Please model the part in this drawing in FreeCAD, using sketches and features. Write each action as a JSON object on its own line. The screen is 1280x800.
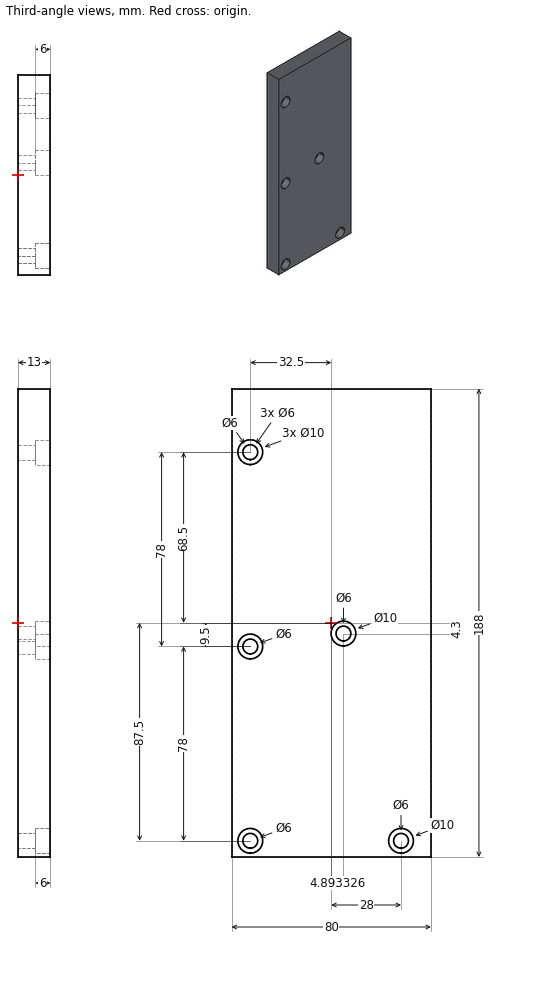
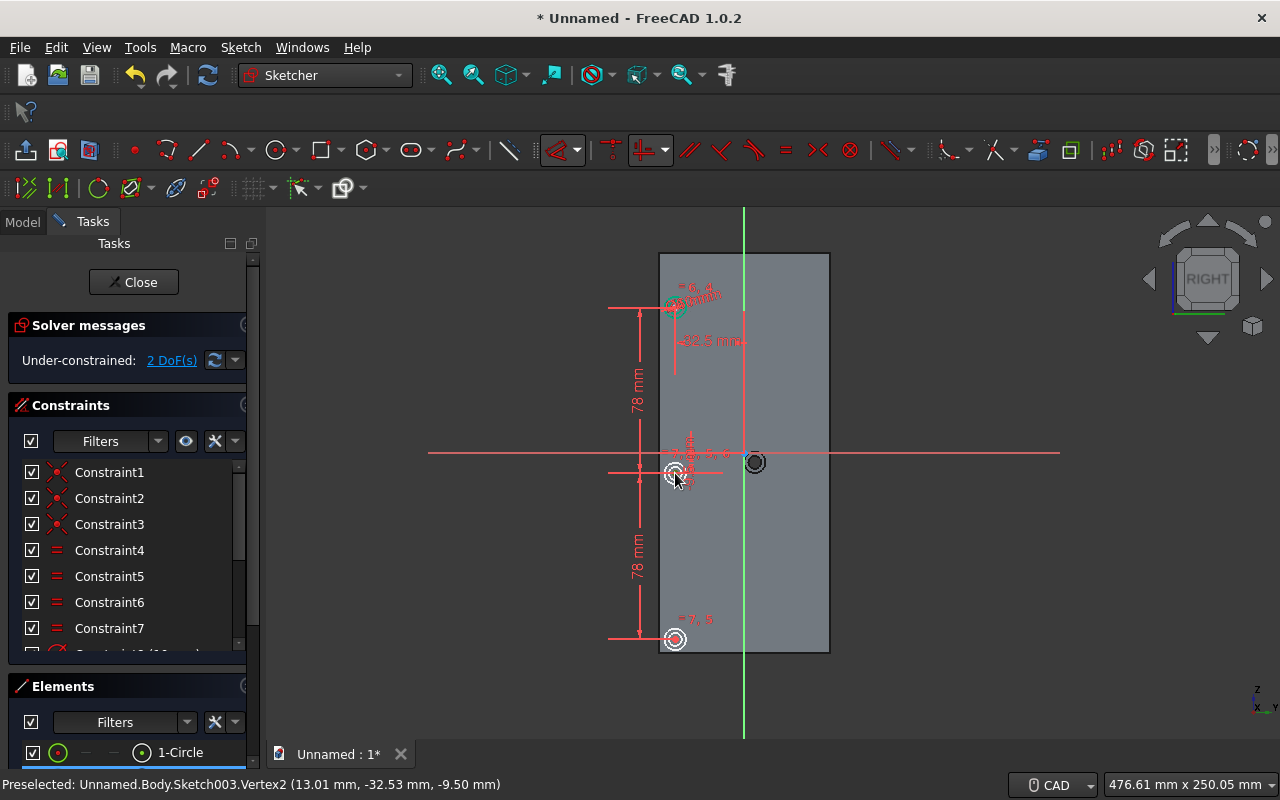
{"action": "left_click", "coordinate": [580, 150]}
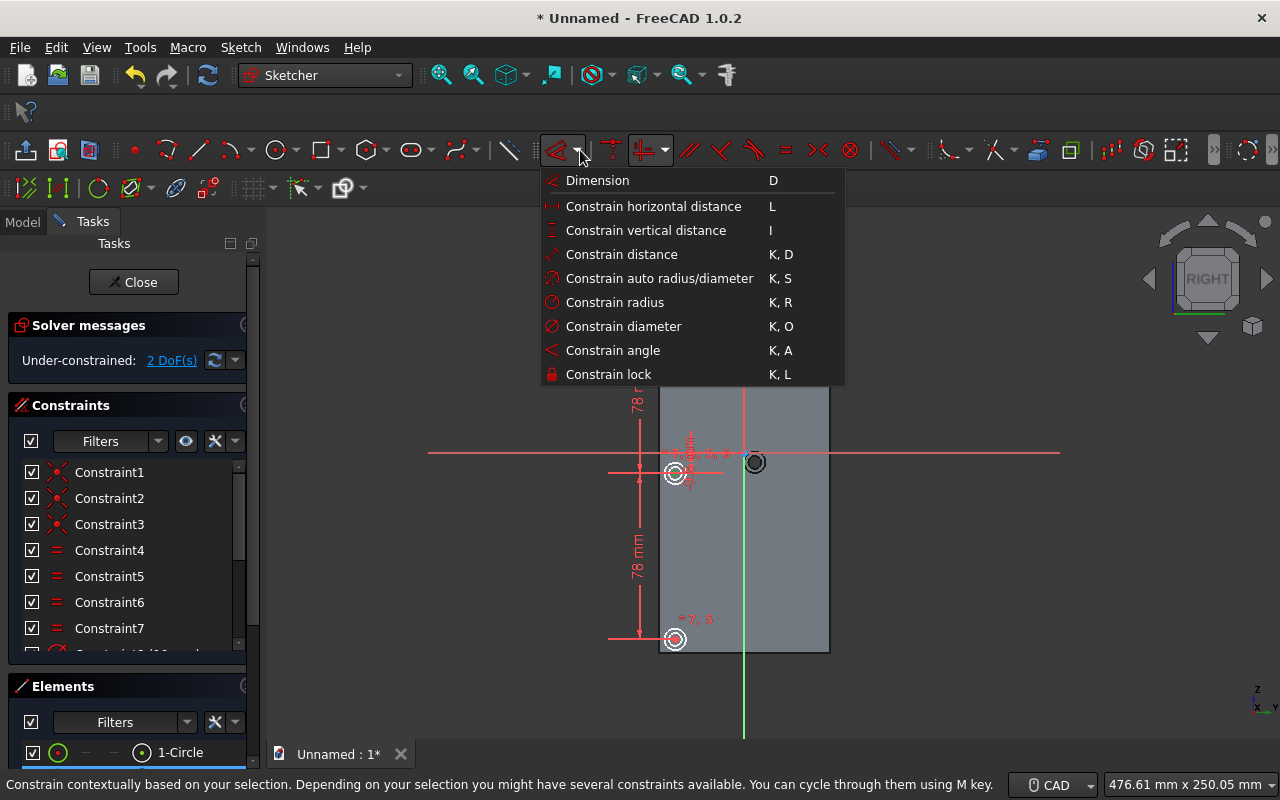
{"action": "left_click", "coordinate": [693, 206]}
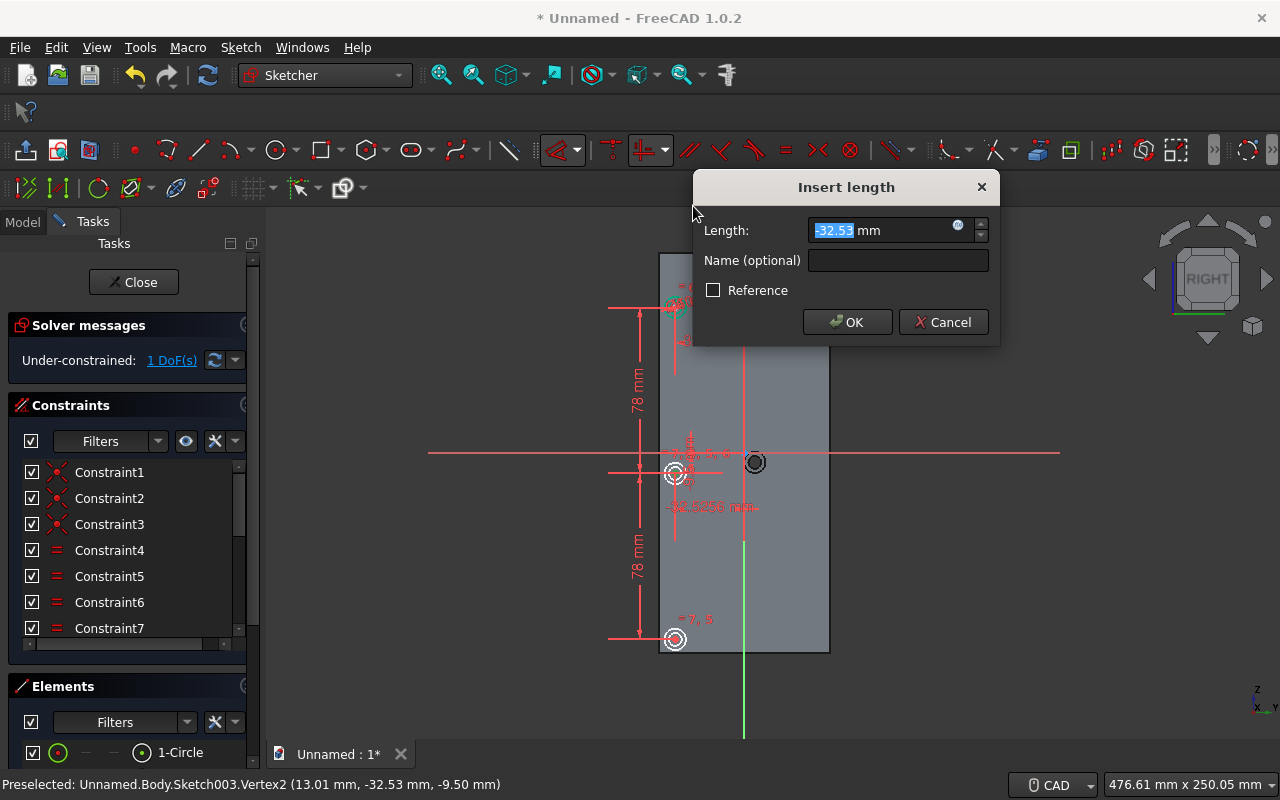
{"action": "type", "text": "-32.5"}
{"action": "key", "text": "Return"}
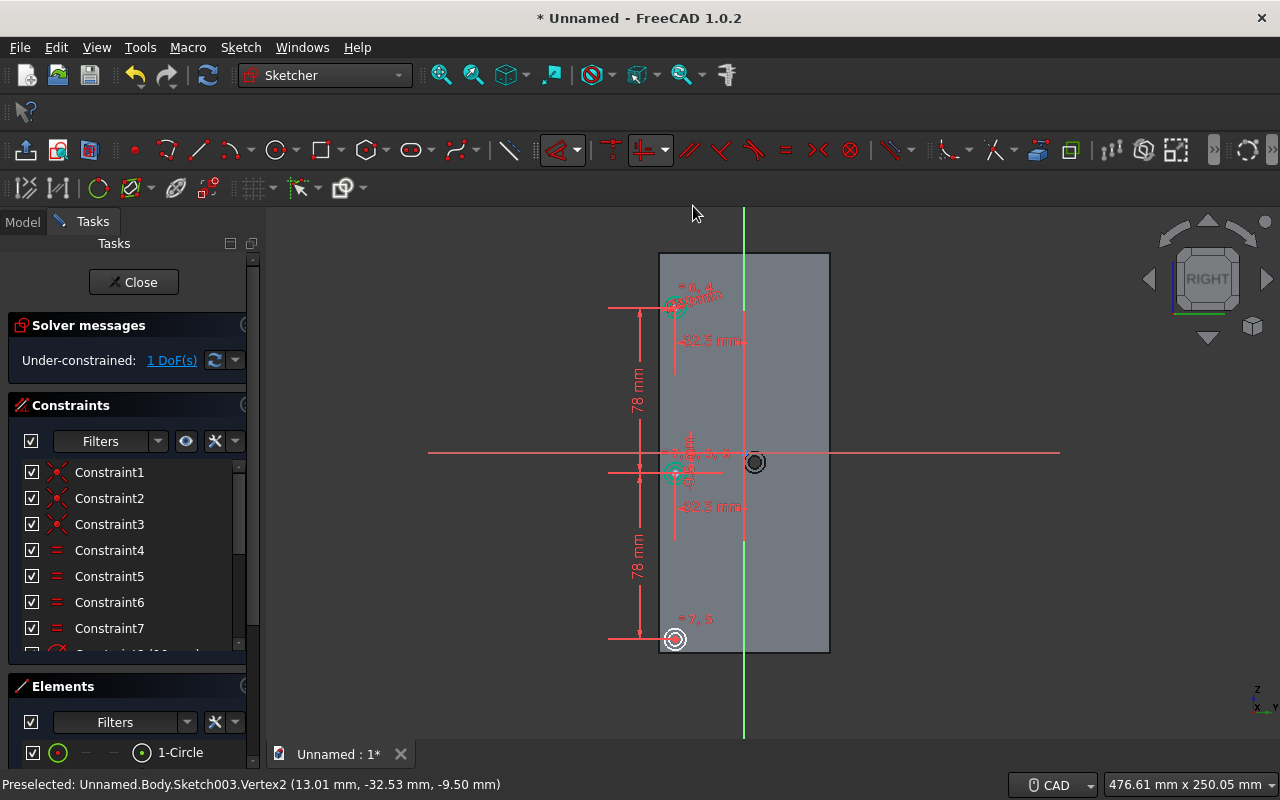
{"action": "left_click", "coordinate": [675, 639]}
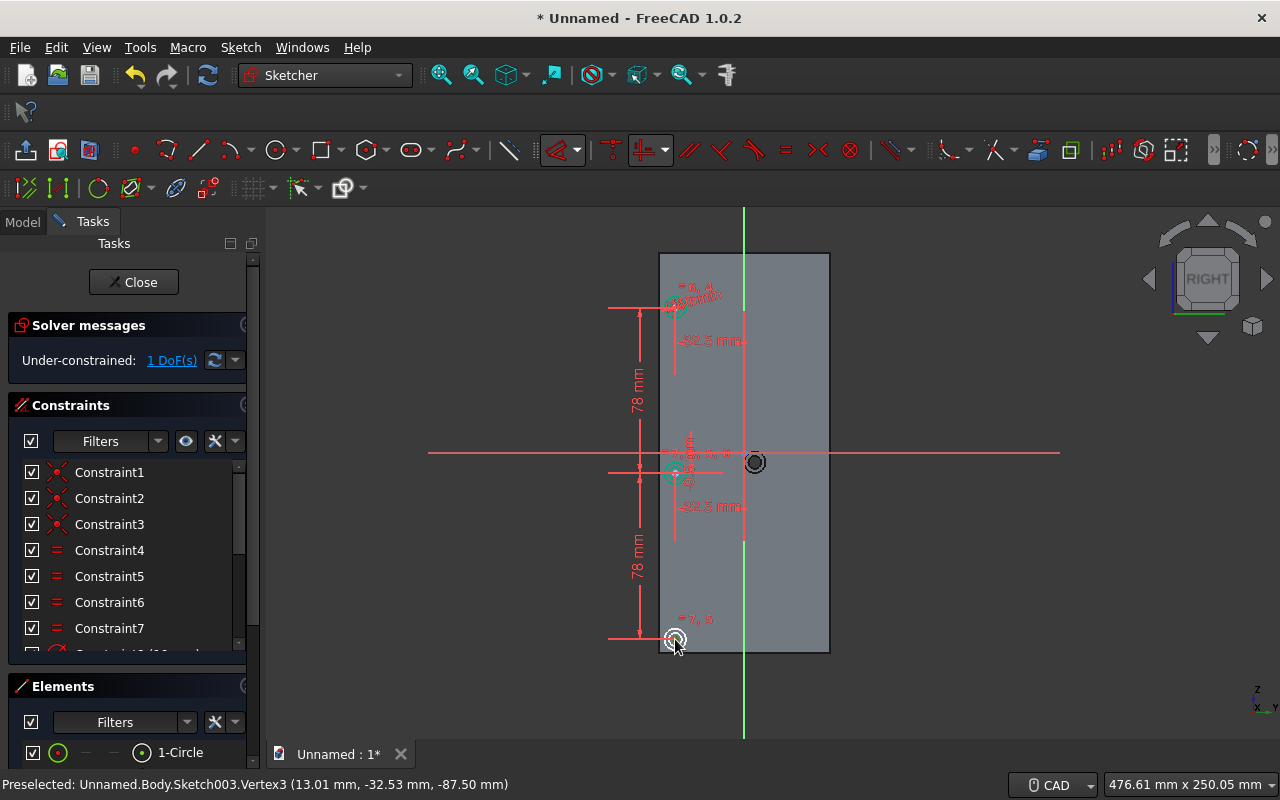
{"action": "key", "text": "l"}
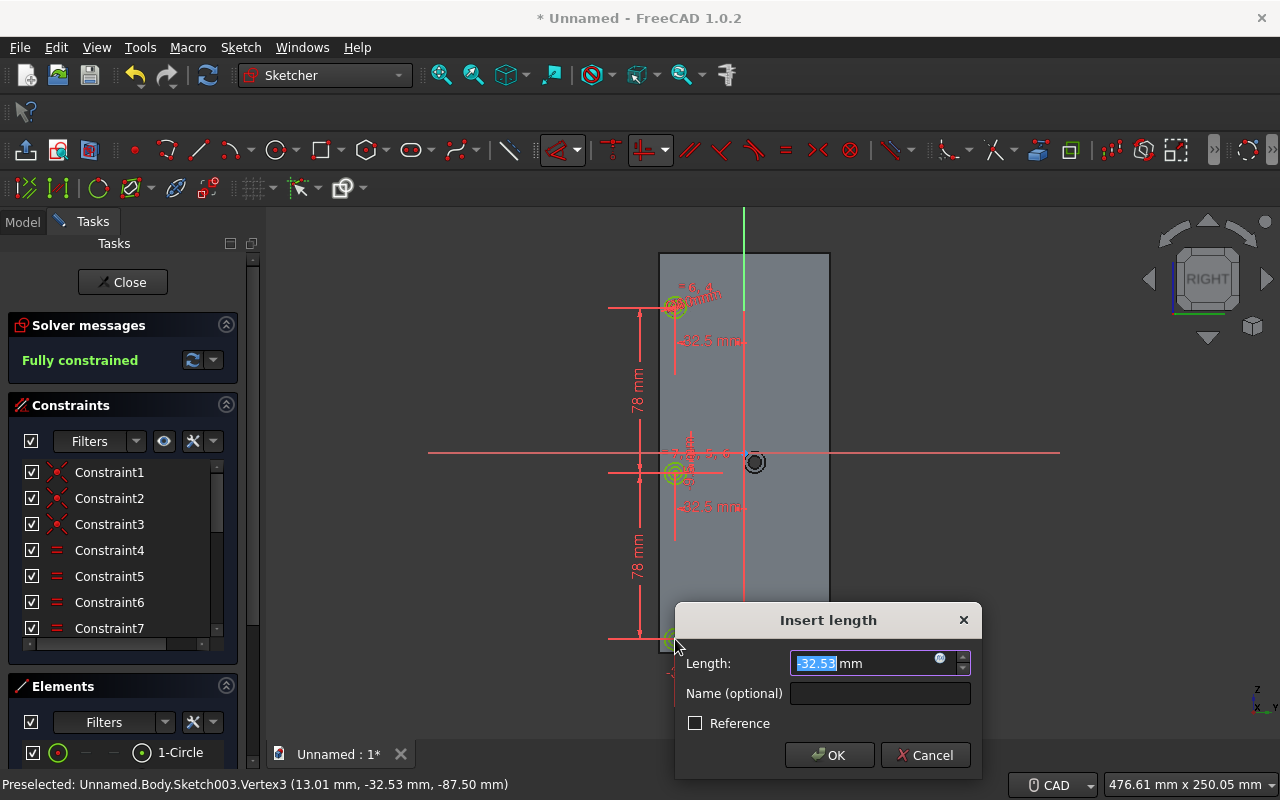
{"action": "type", "text": "-32.5"}
{"action": "key", "text": "Return"}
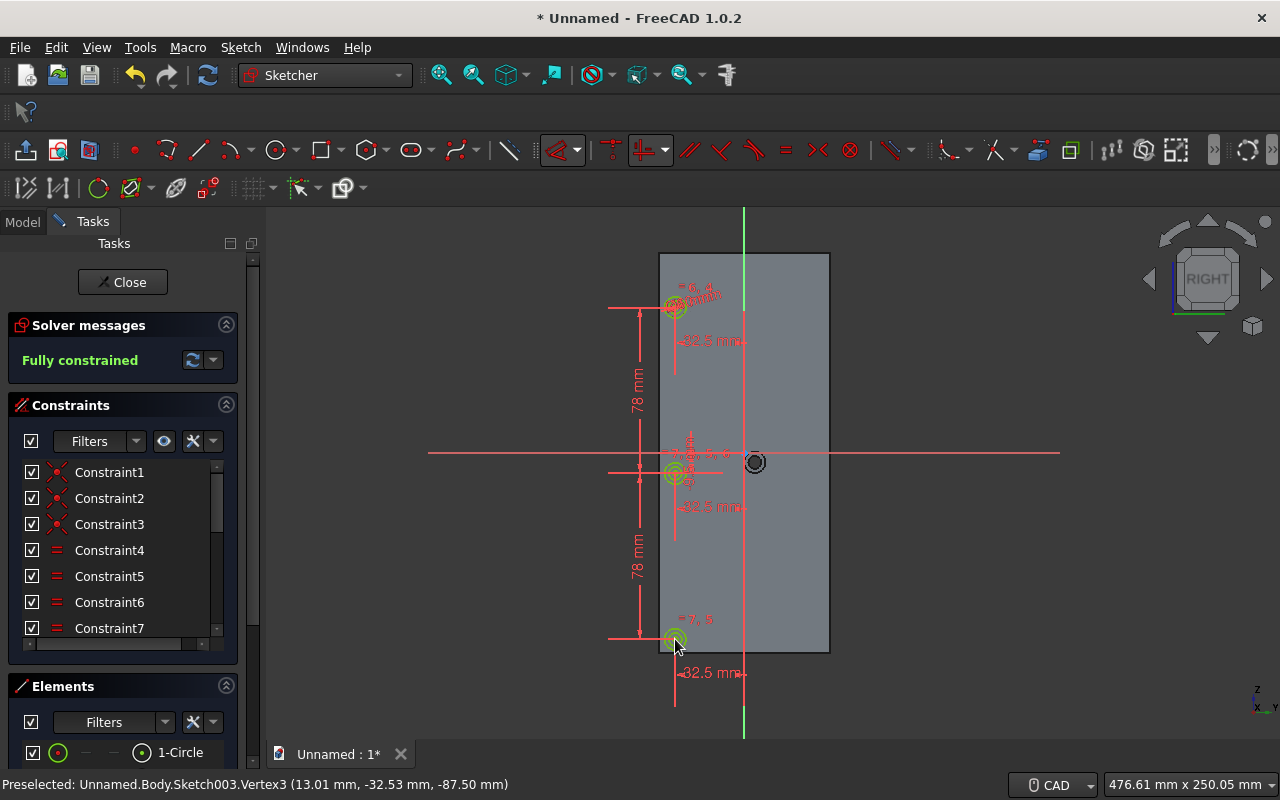
{"action": "left_click", "coordinate": [123, 282]}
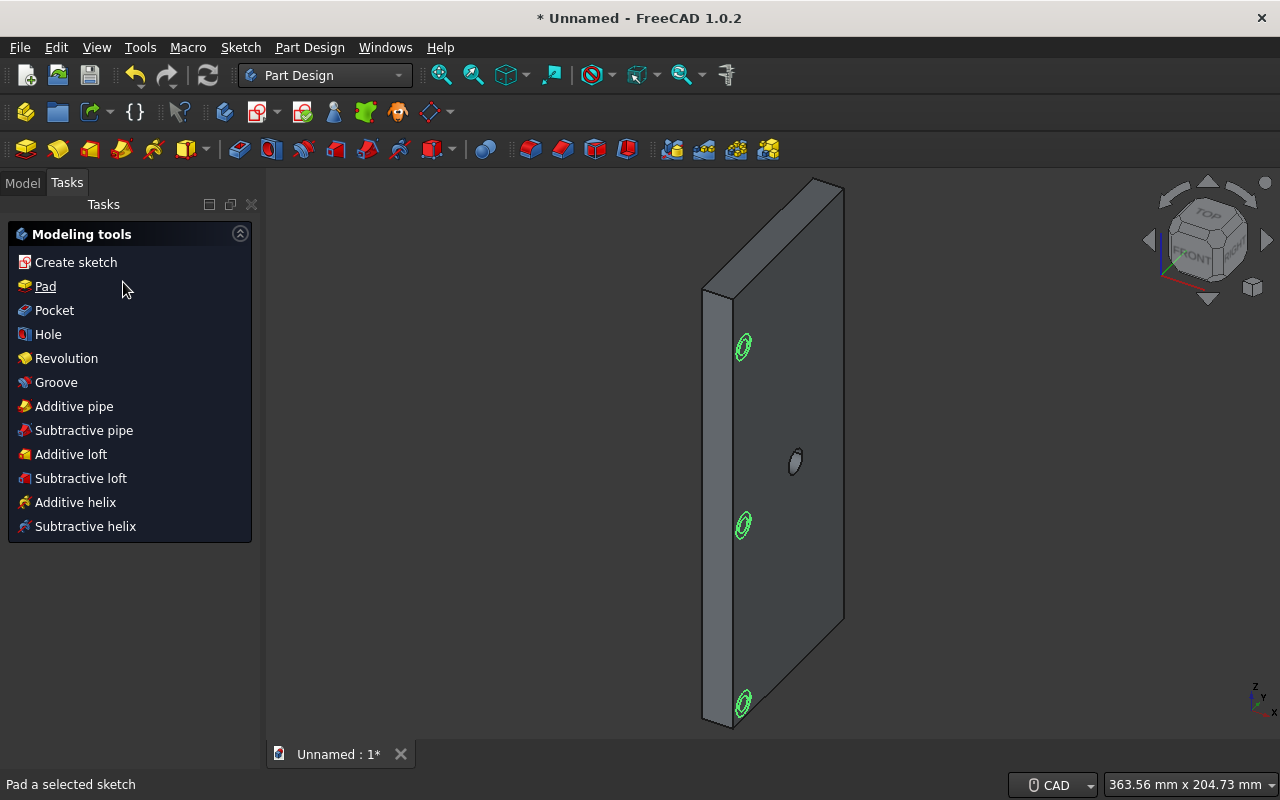
{"action": "left_click", "coordinate": [240, 150]}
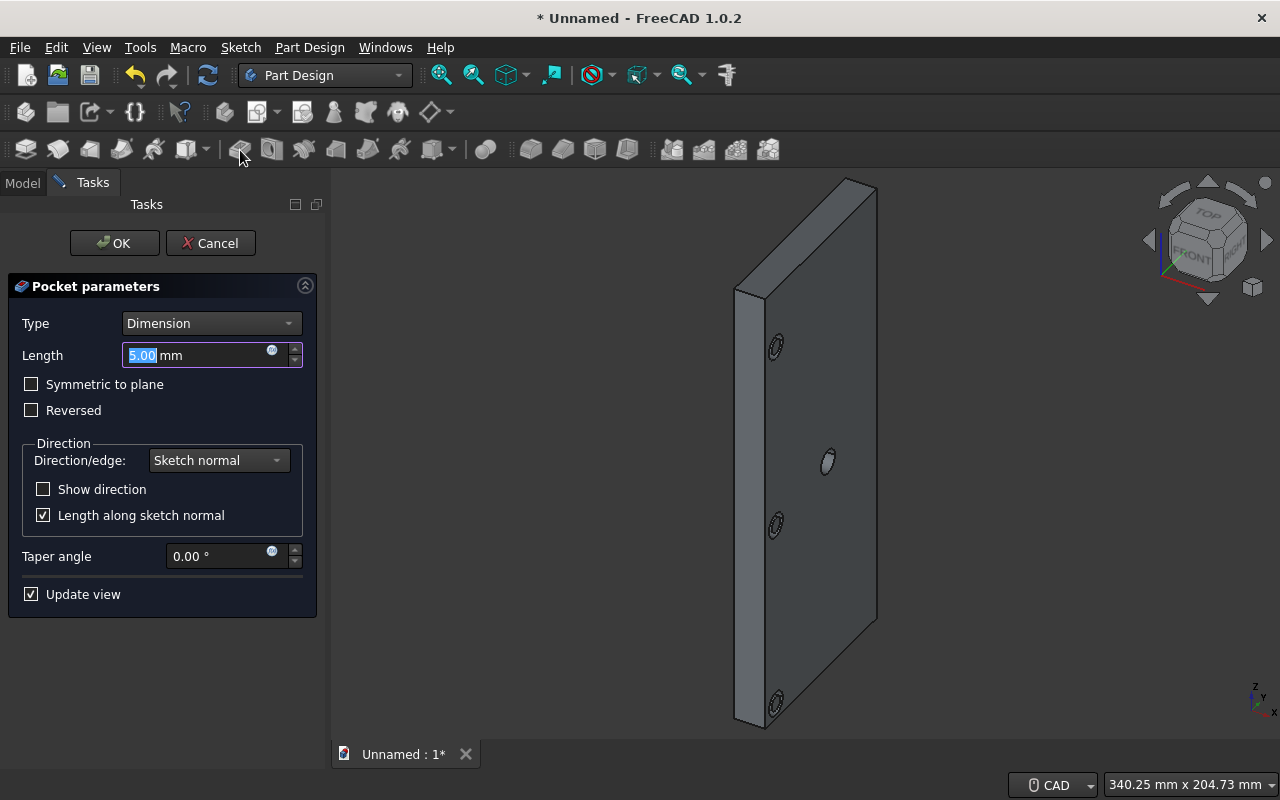
{"action": "type", "text": "6"}
{"action": "key", "text": "Tab"}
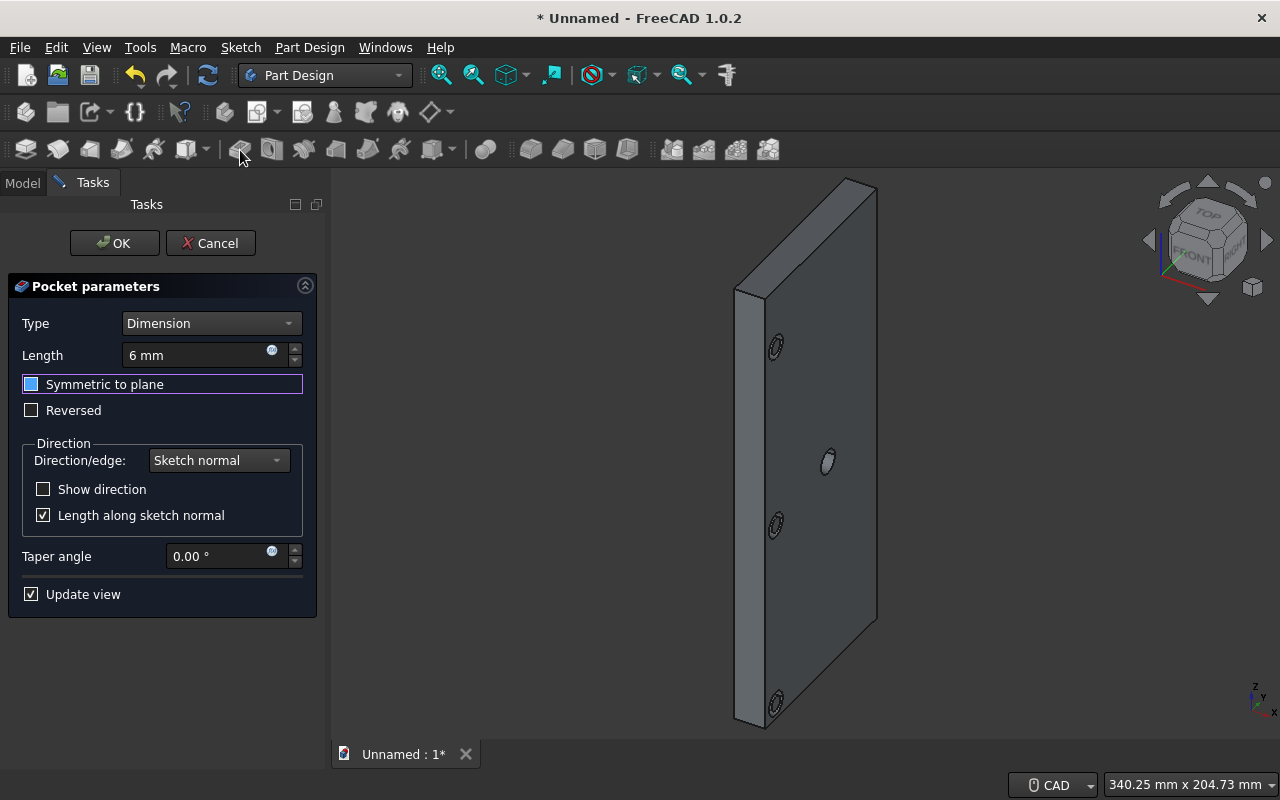
{"action": "left_click", "coordinate": [115, 243]}